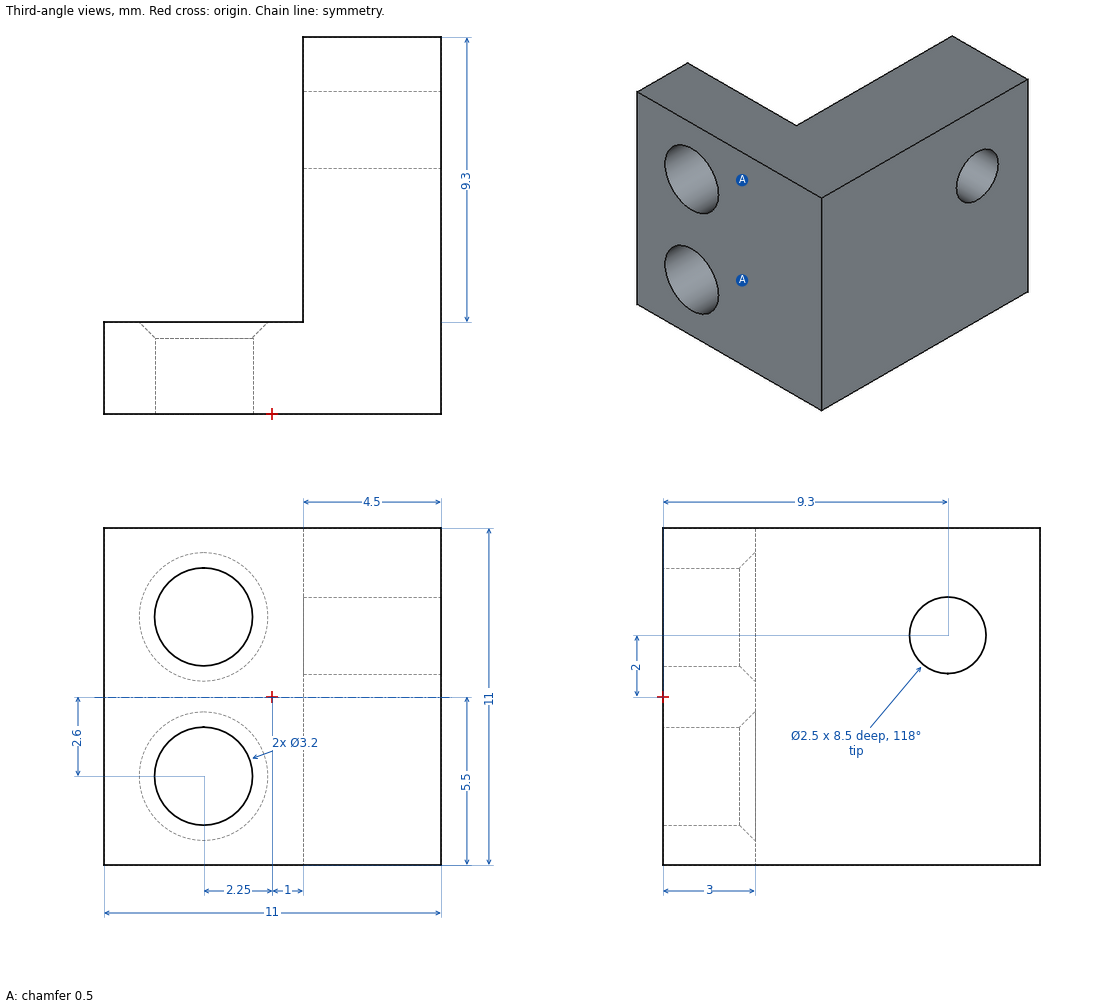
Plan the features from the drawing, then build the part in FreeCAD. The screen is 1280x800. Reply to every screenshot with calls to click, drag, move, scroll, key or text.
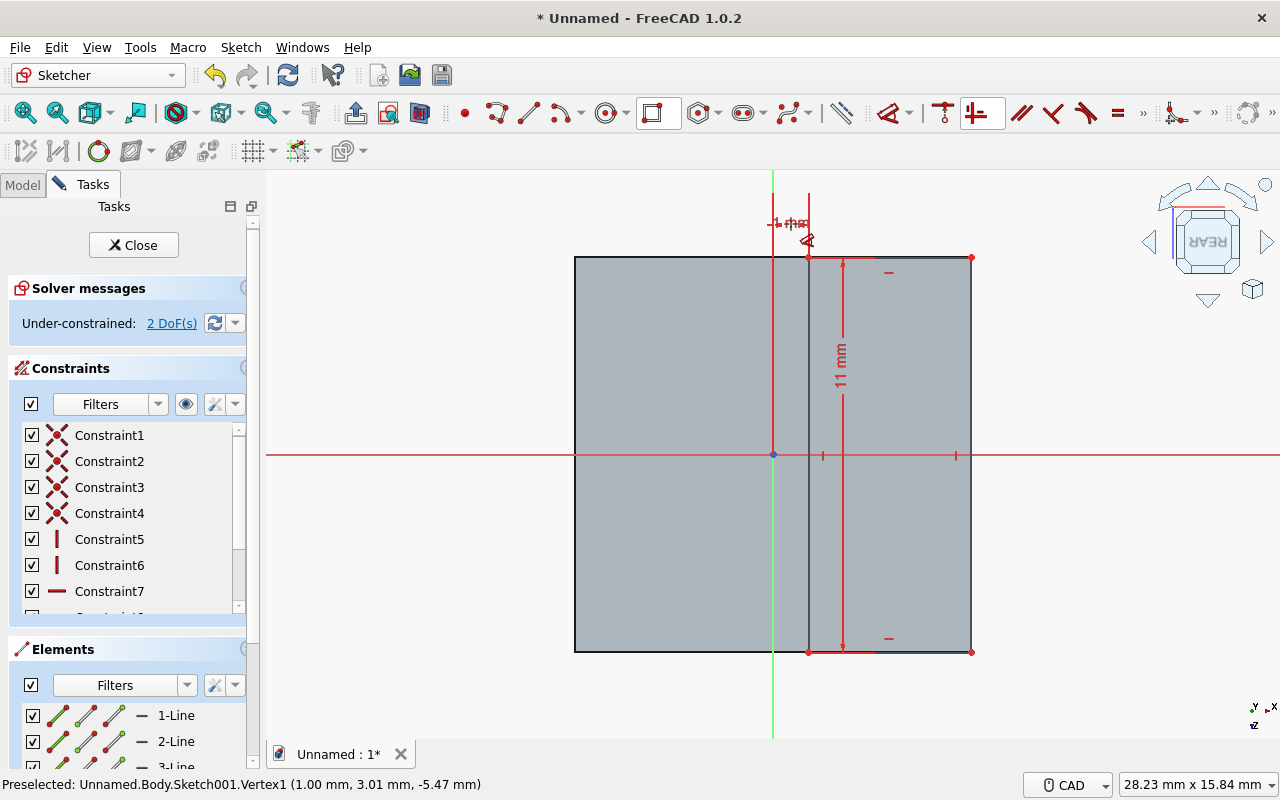
click(858, 653)
click(890, 687)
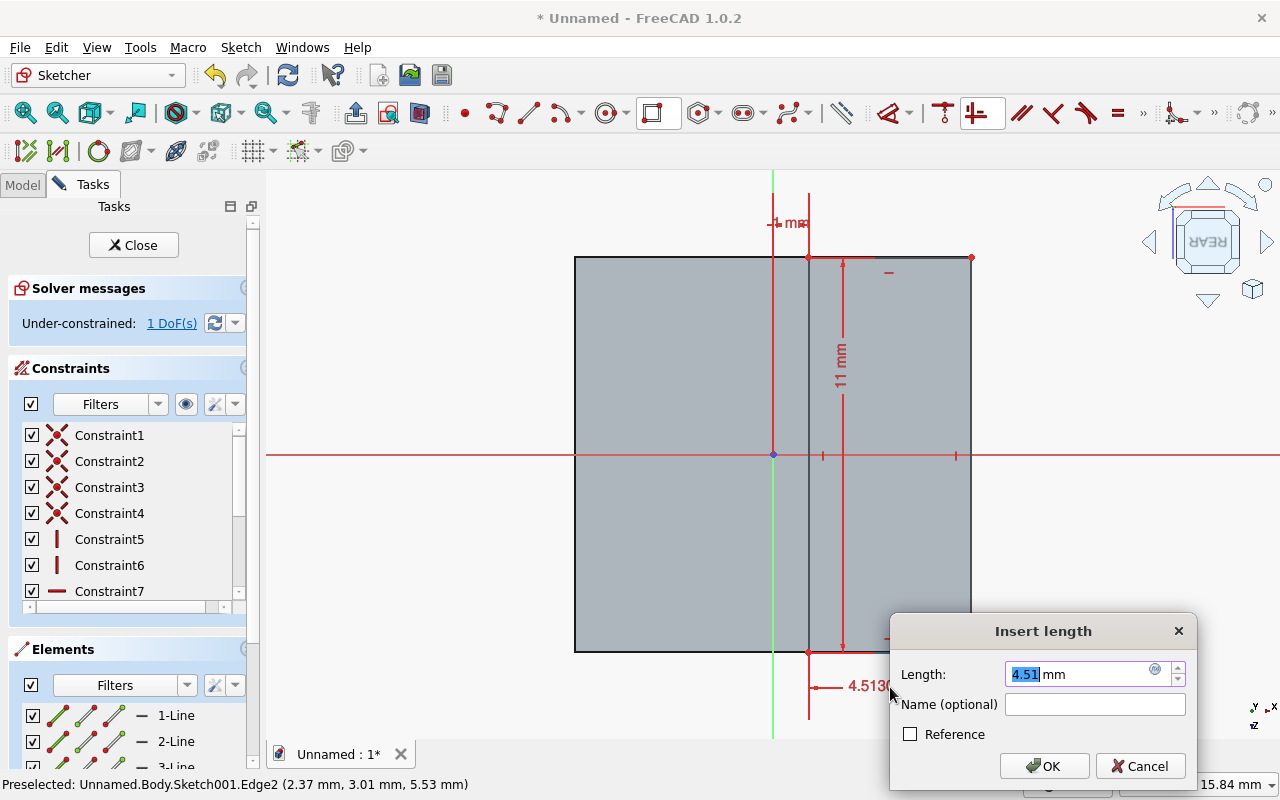
text(4.5)
key(Return)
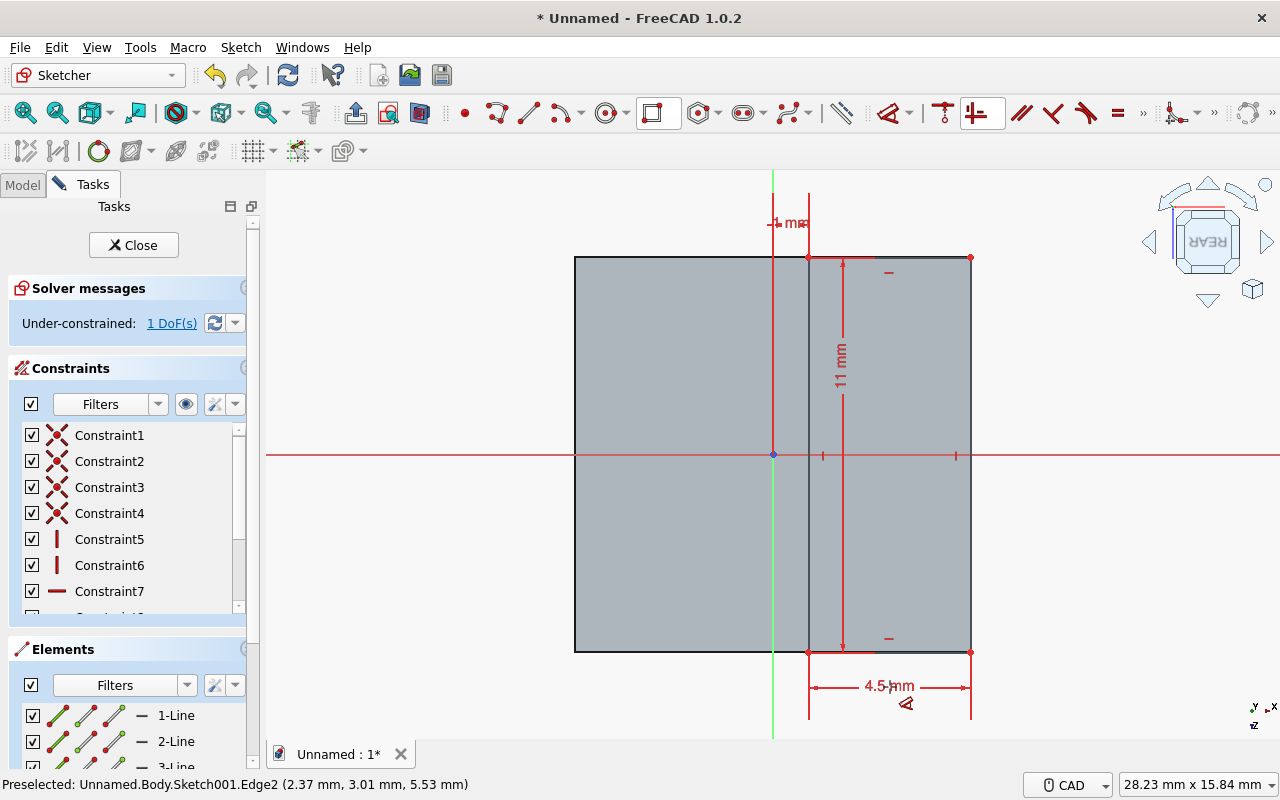
click(809, 258)
click(739, 356)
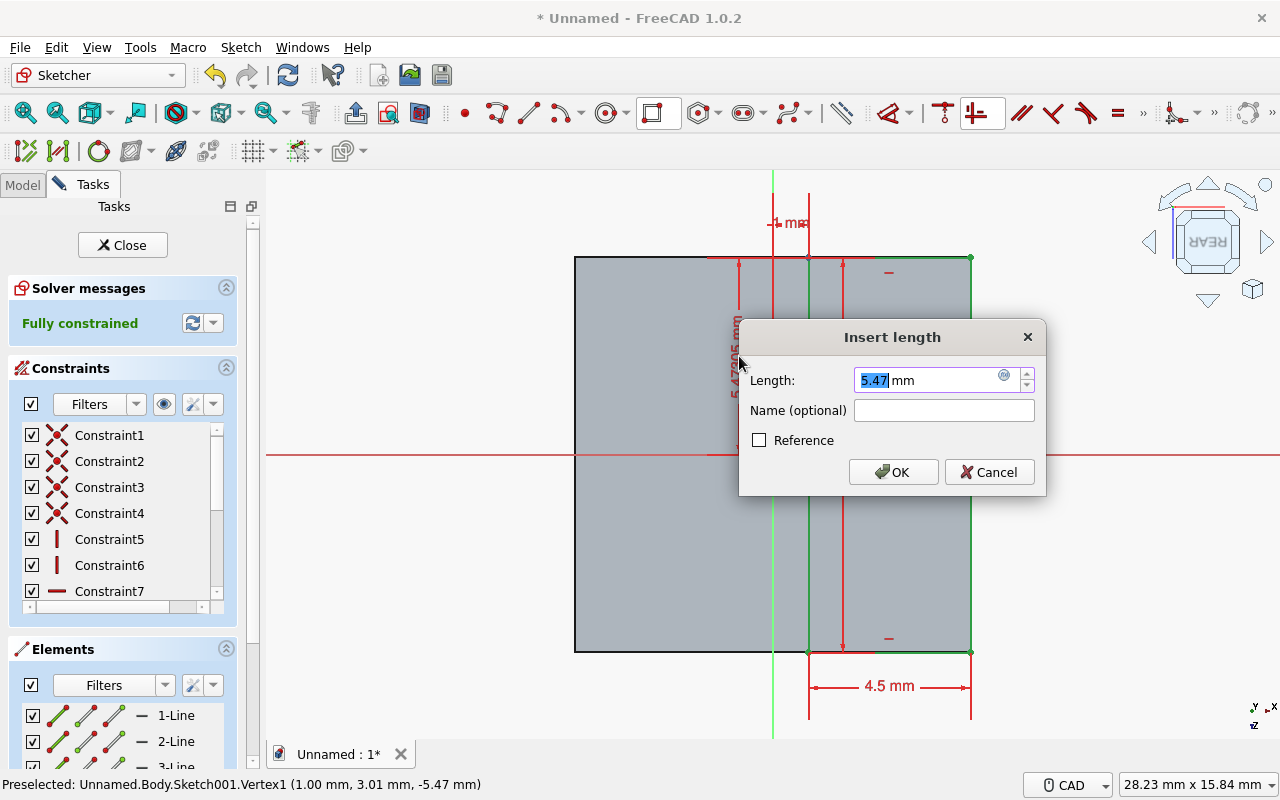
text(5.5)
key(Return)
key(Escape)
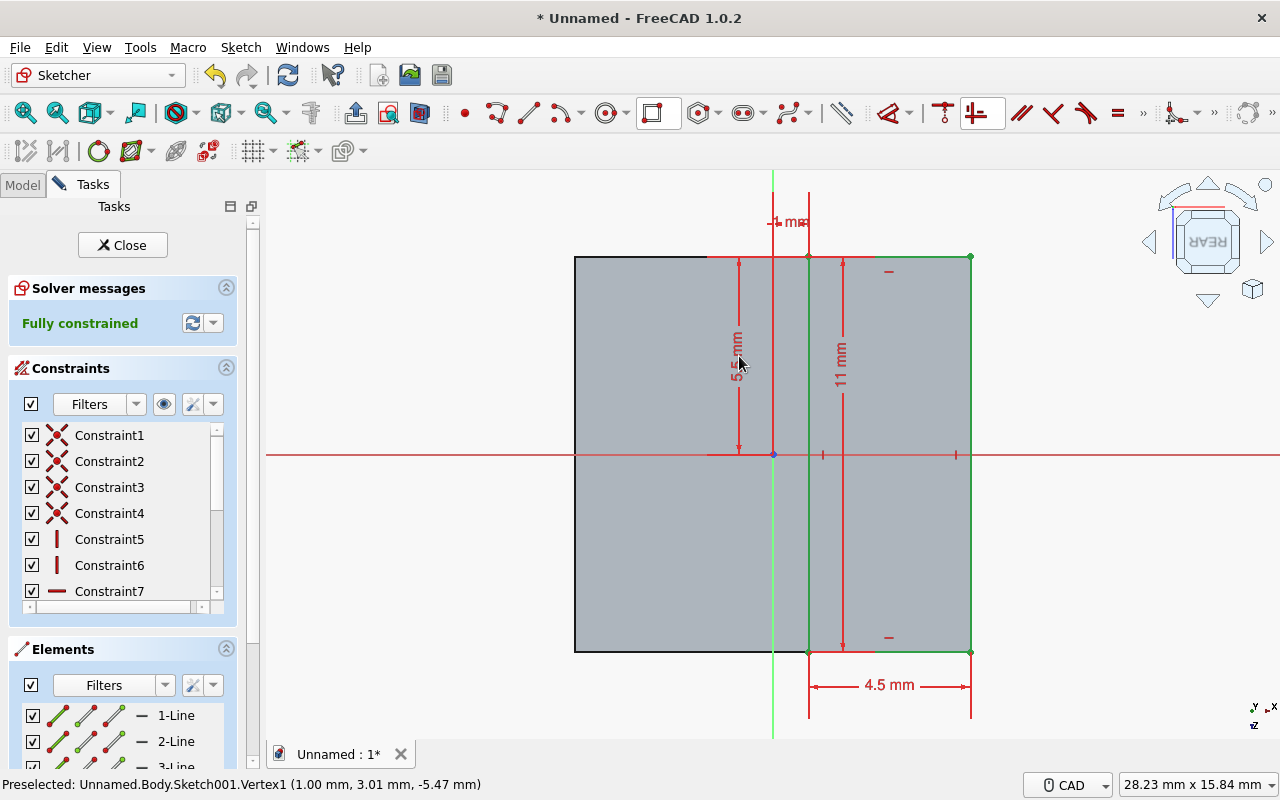
click(123, 245)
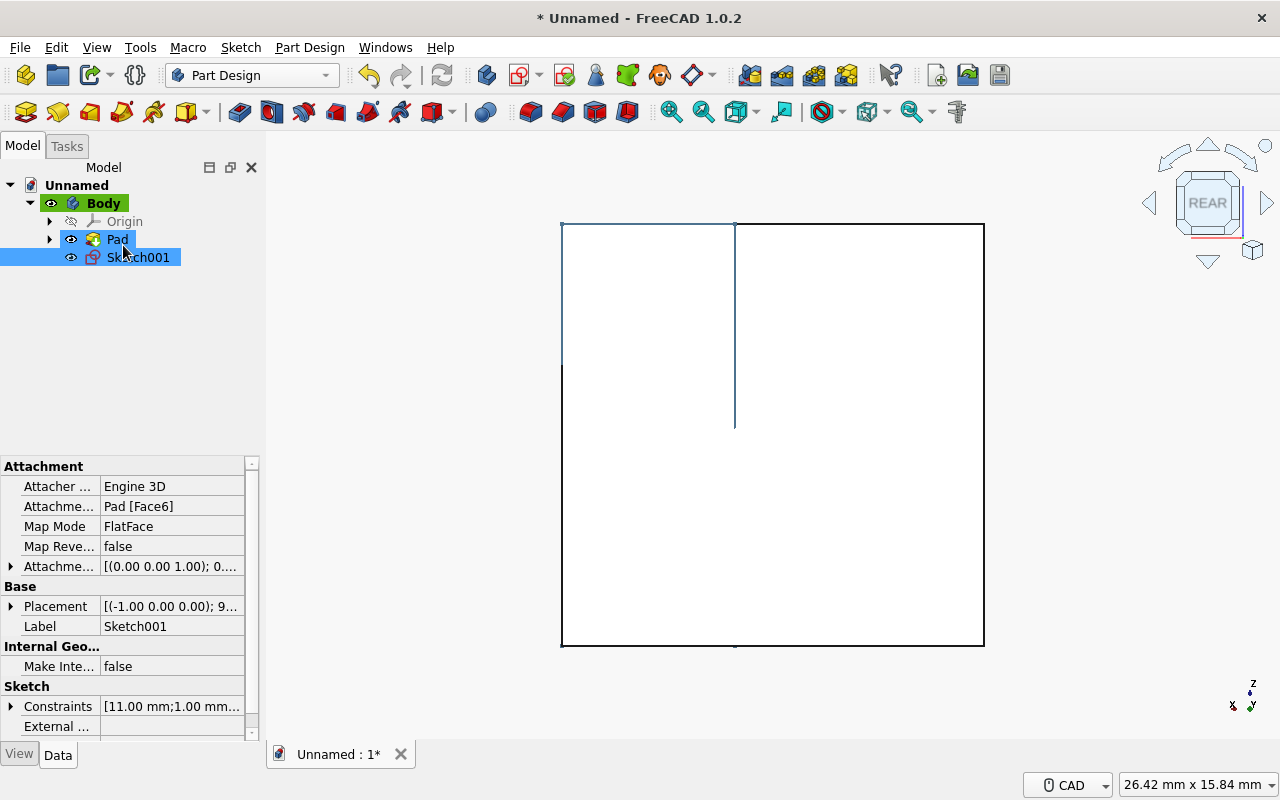
click(26, 112)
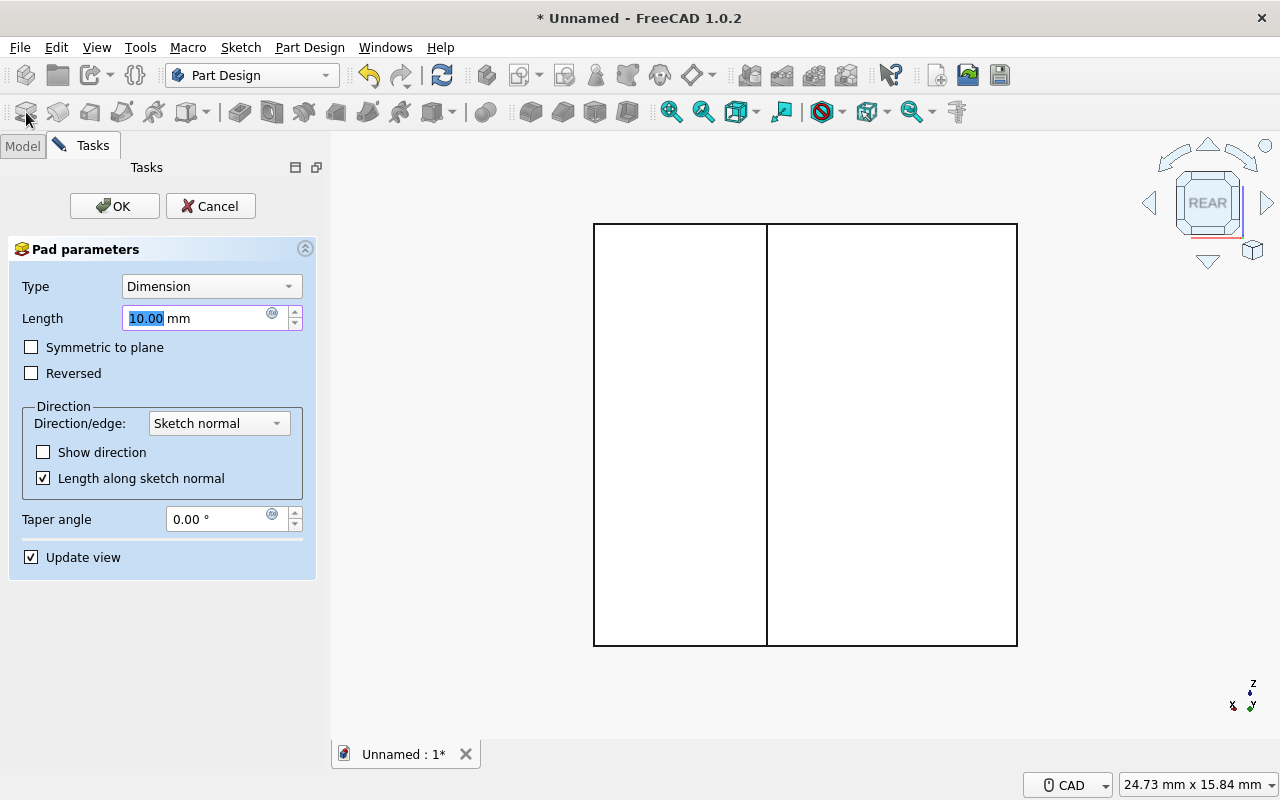
text(9.3)
key(Tab)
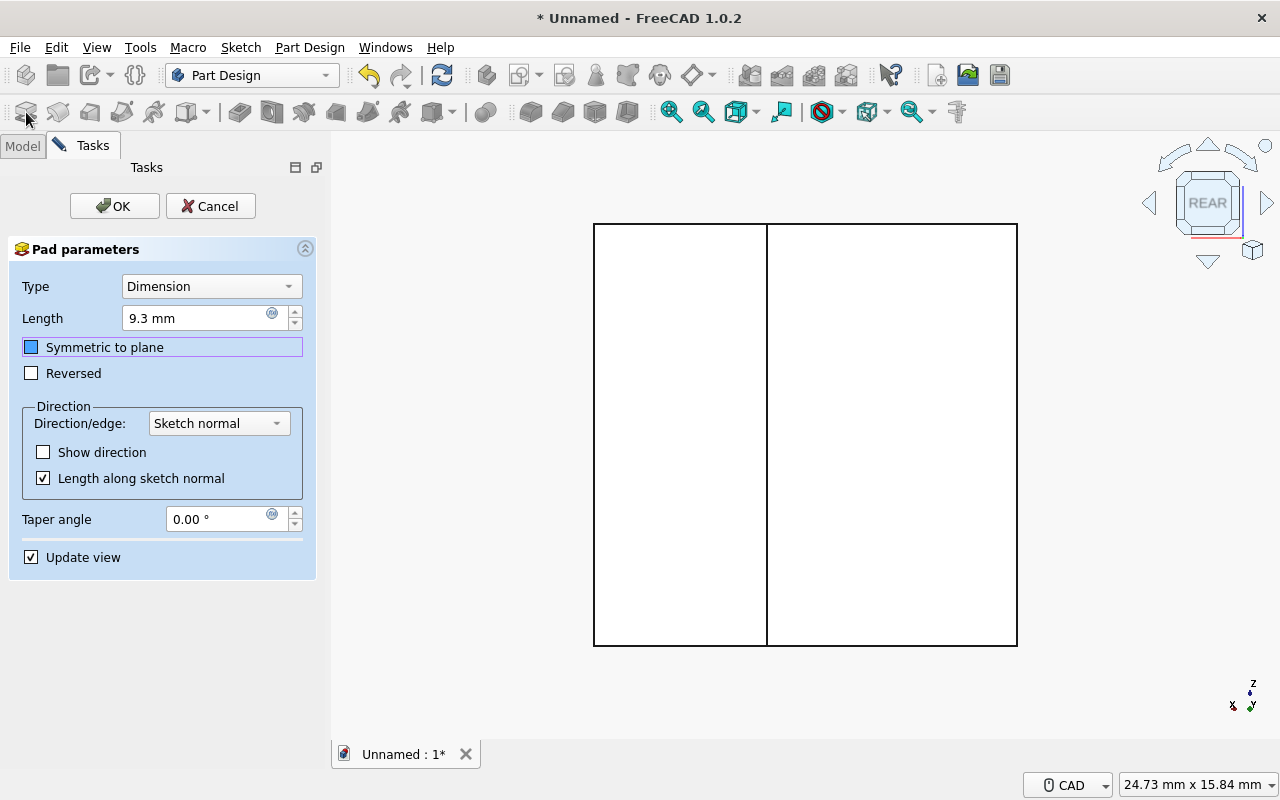
click(115, 206)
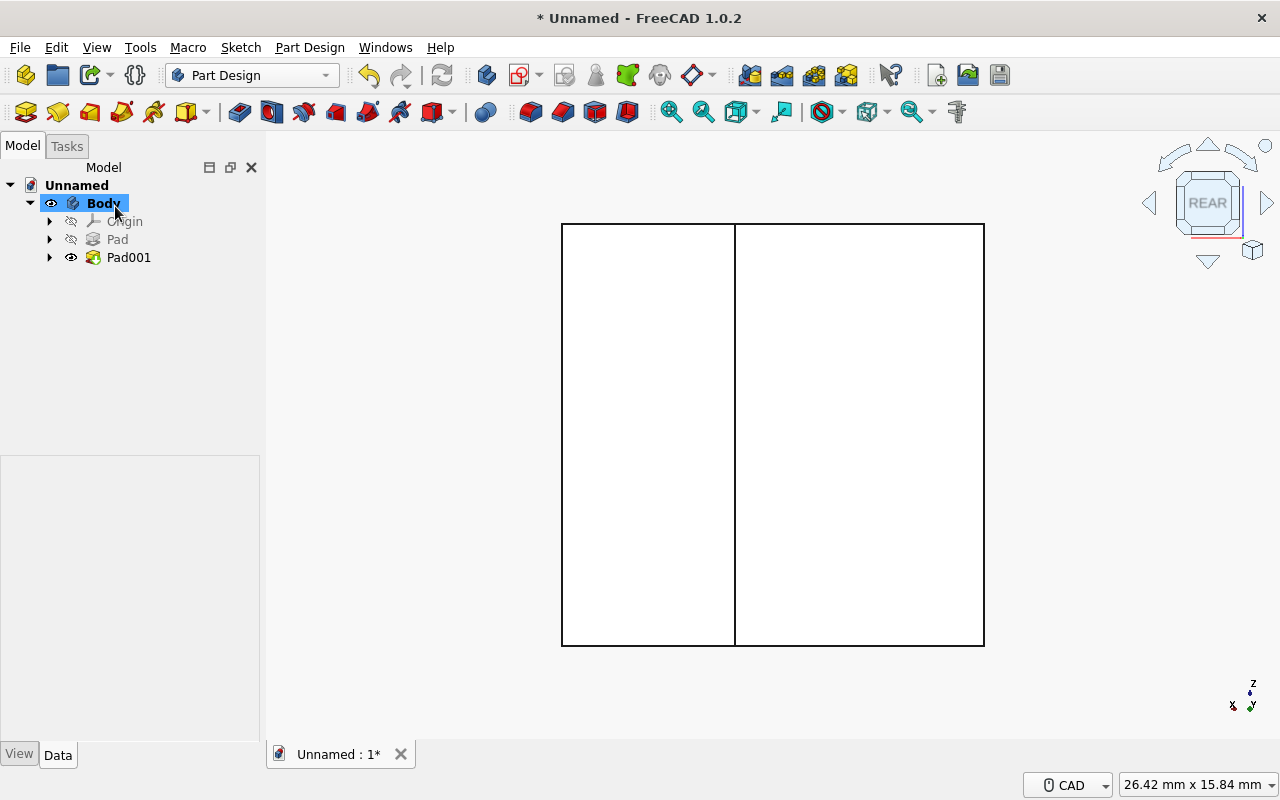
key(6)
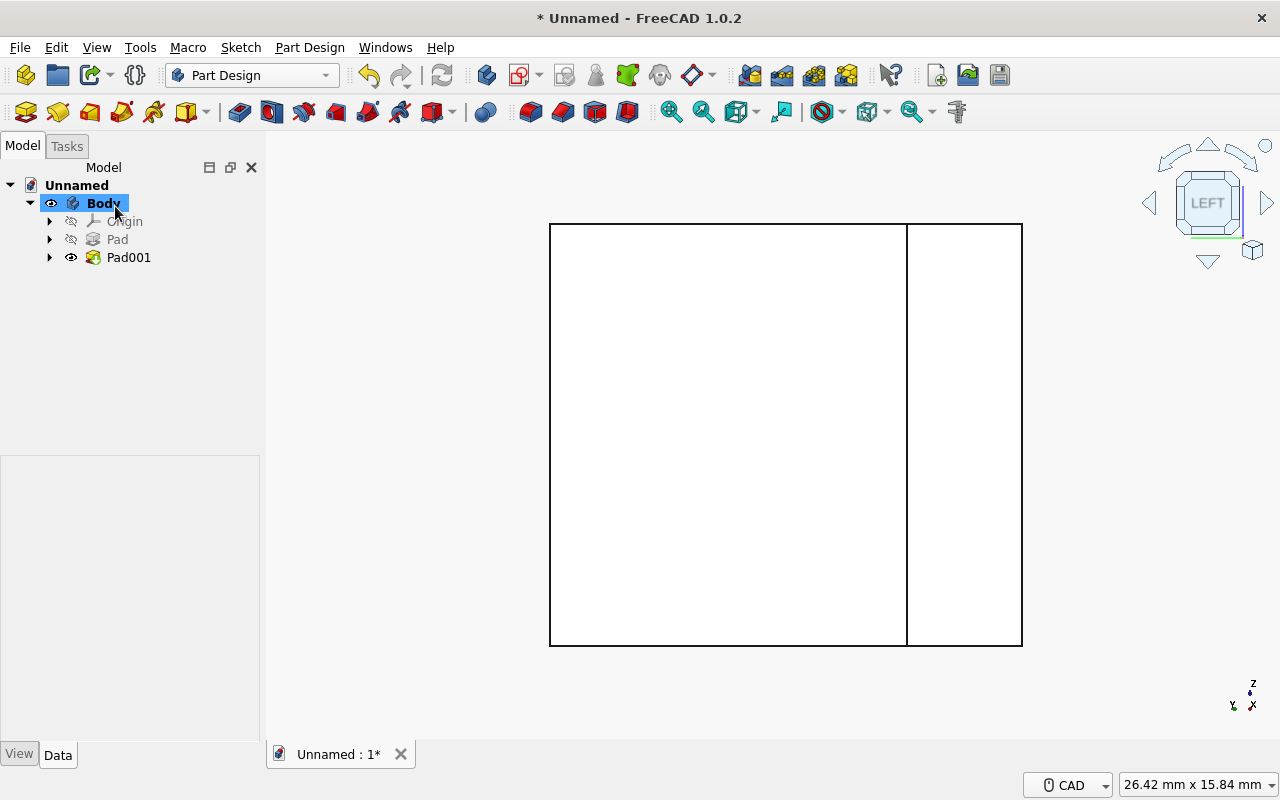
click(729, 434)